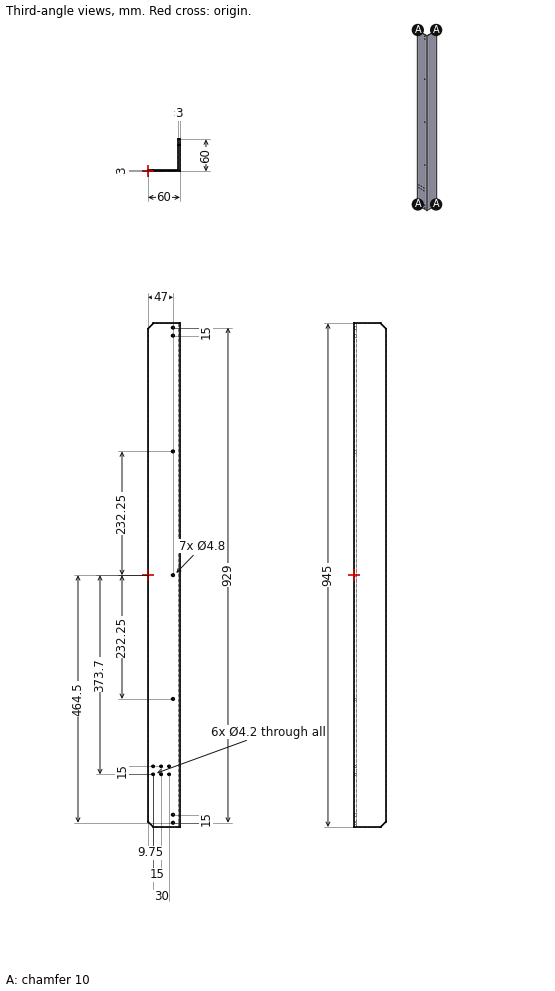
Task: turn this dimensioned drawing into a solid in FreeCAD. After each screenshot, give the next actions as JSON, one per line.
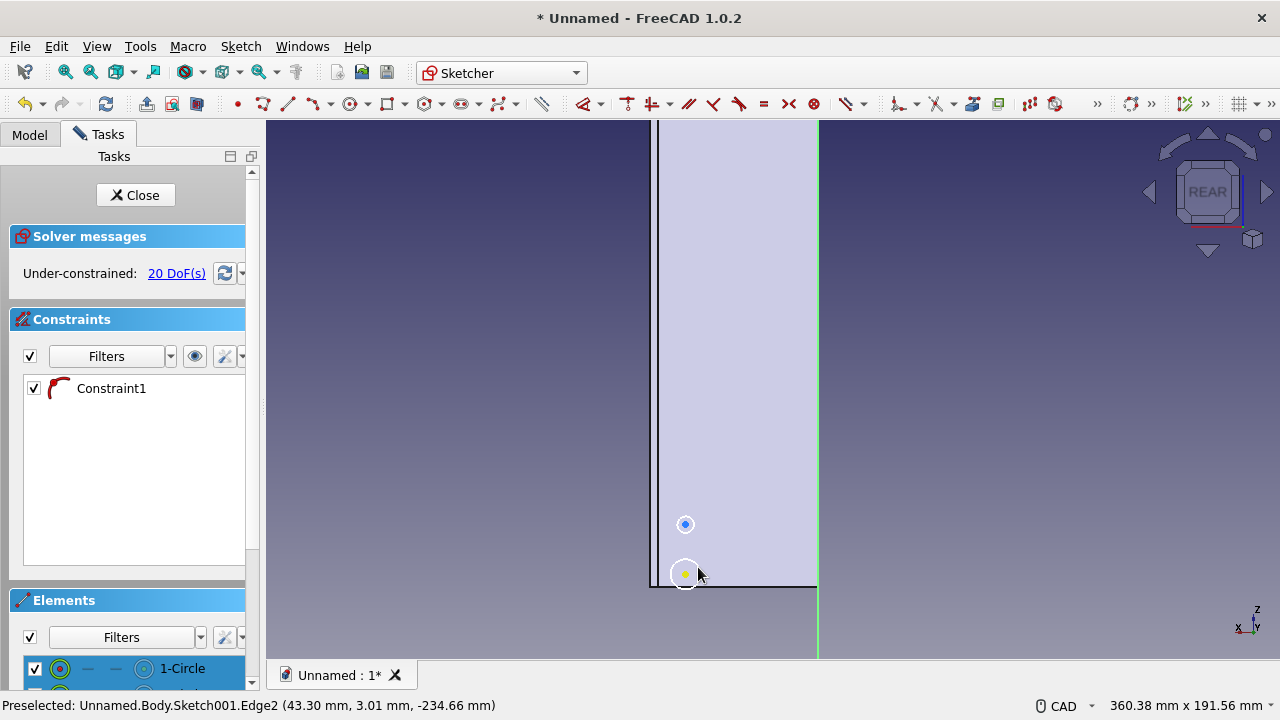
{"action": "left_click", "coordinate": [696, 564]}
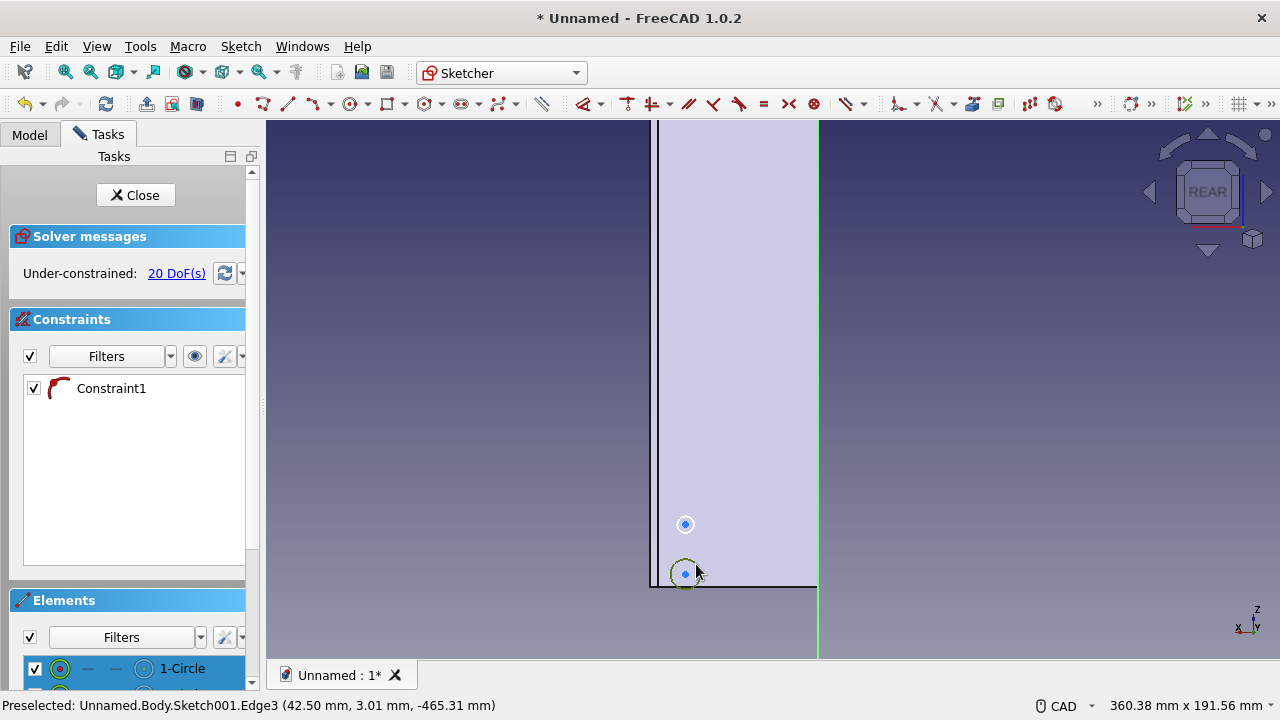
{"action": "scroll", "coordinate": [698, 567], "scroll_direction": "down", "scroll_amount": 10}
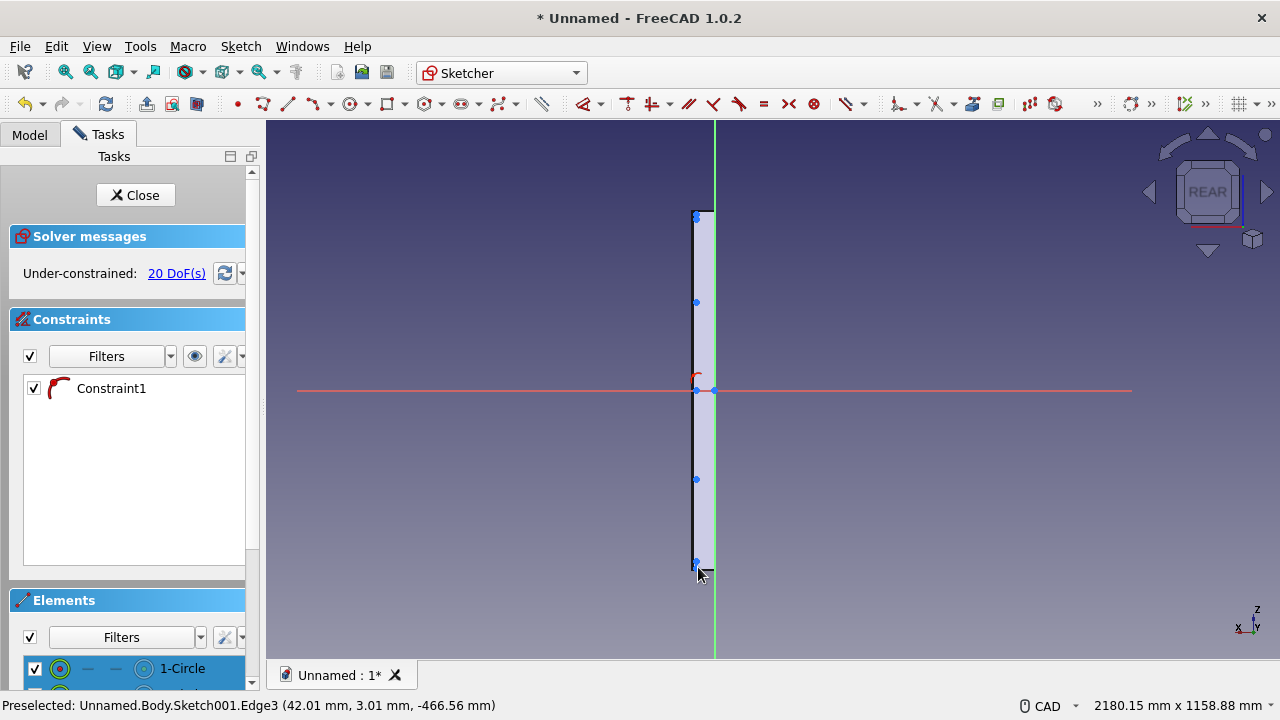
{"action": "scroll", "coordinate": [698, 213], "scroll_direction": "up", "scroll_amount": 11}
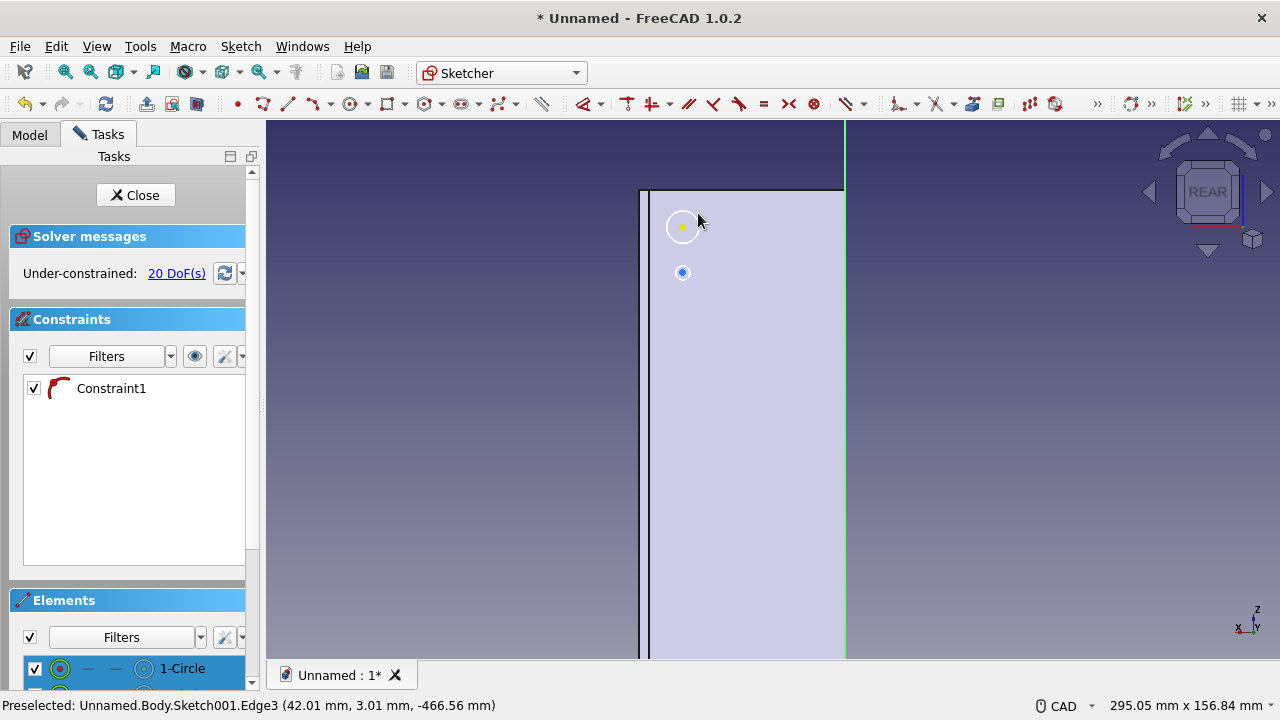
{"action": "left_click", "coordinate": [694, 216]}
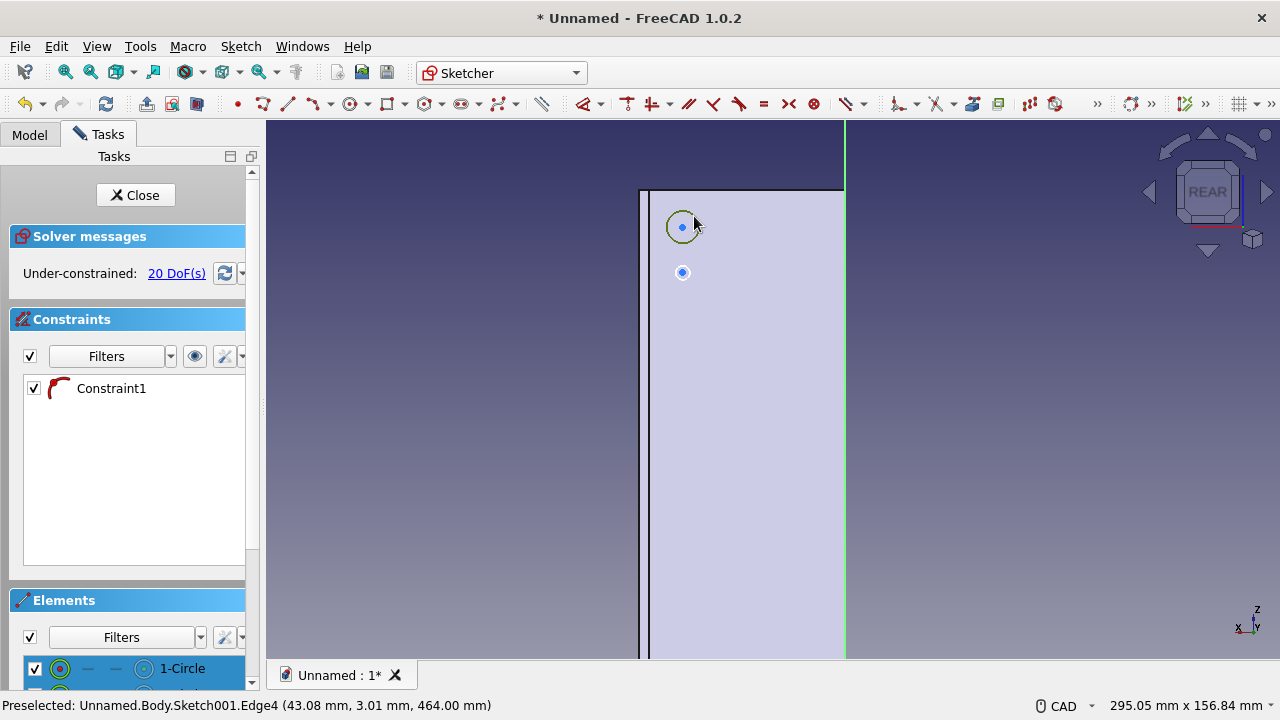
{"action": "scroll", "coordinate": [698, 212], "scroll_direction": "down", "scroll_amount": 11}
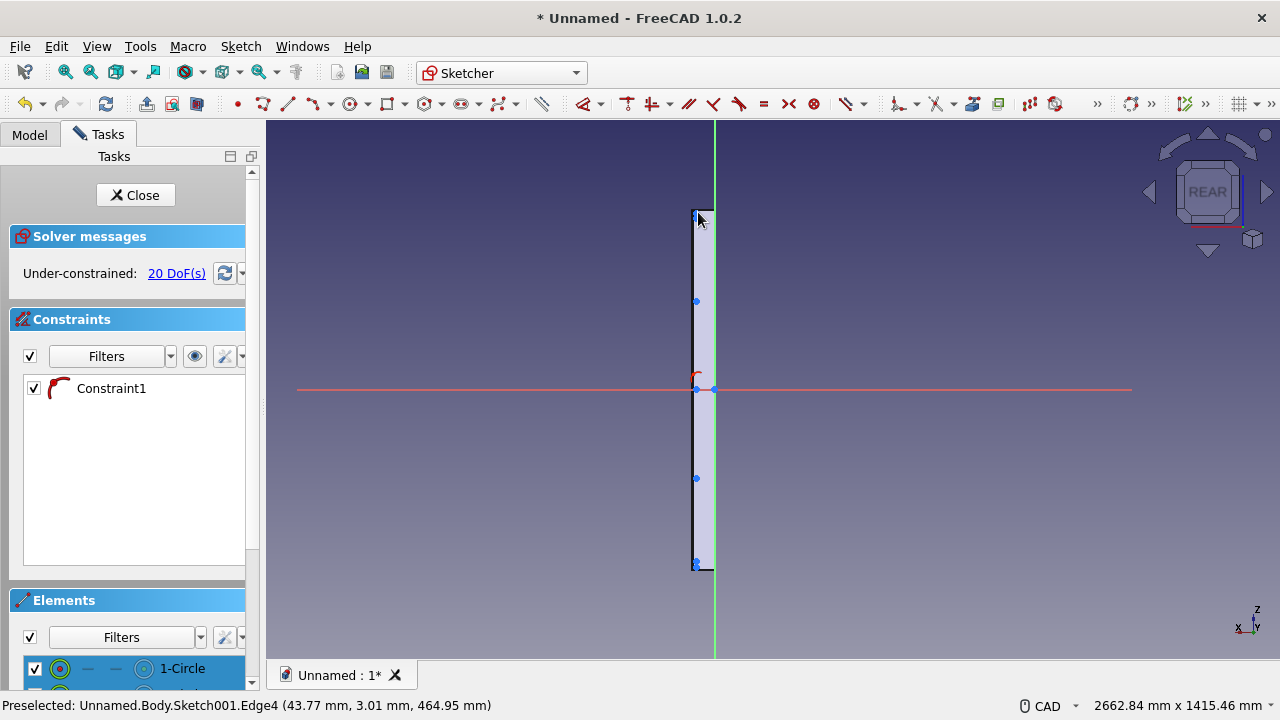
{"action": "scroll", "coordinate": [698, 301], "scroll_direction": "up", "scroll_amount": 12}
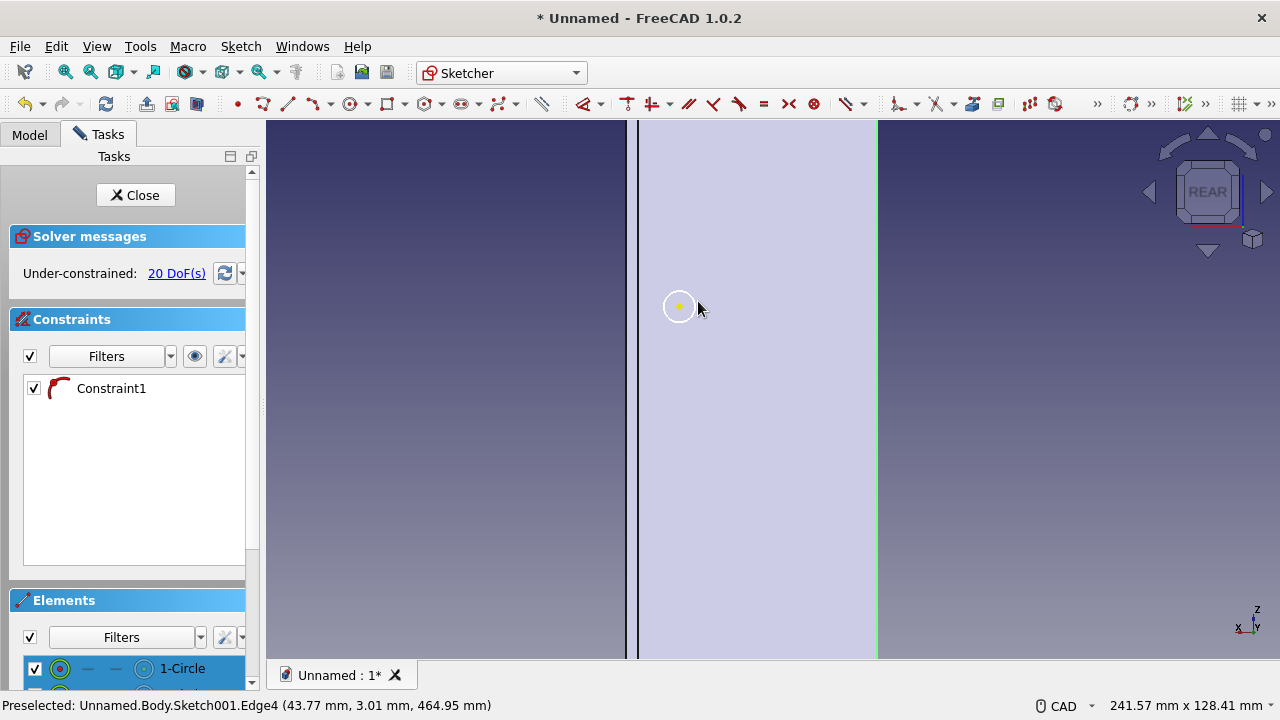
{"action": "left_click", "coordinate": [690, 296]}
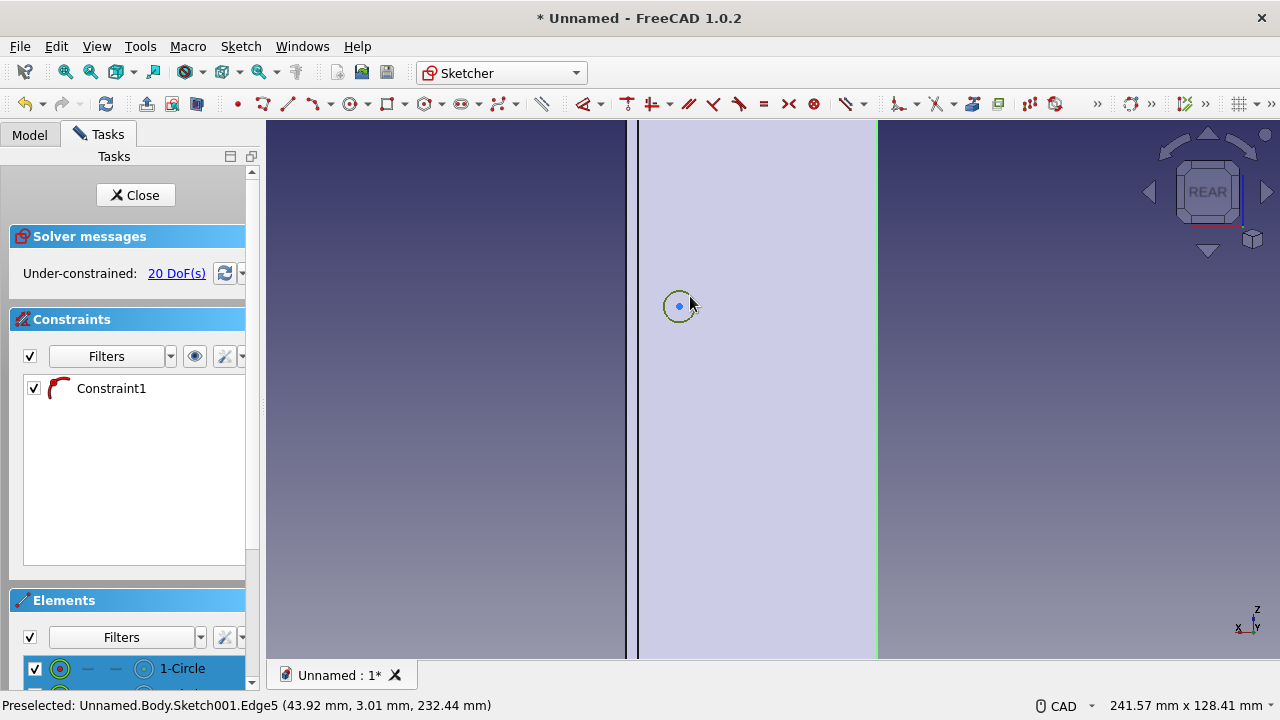
{"action": "scroll", "coordinate": [698, 301], "scroll_direction": "down", "scroll_amount": 12}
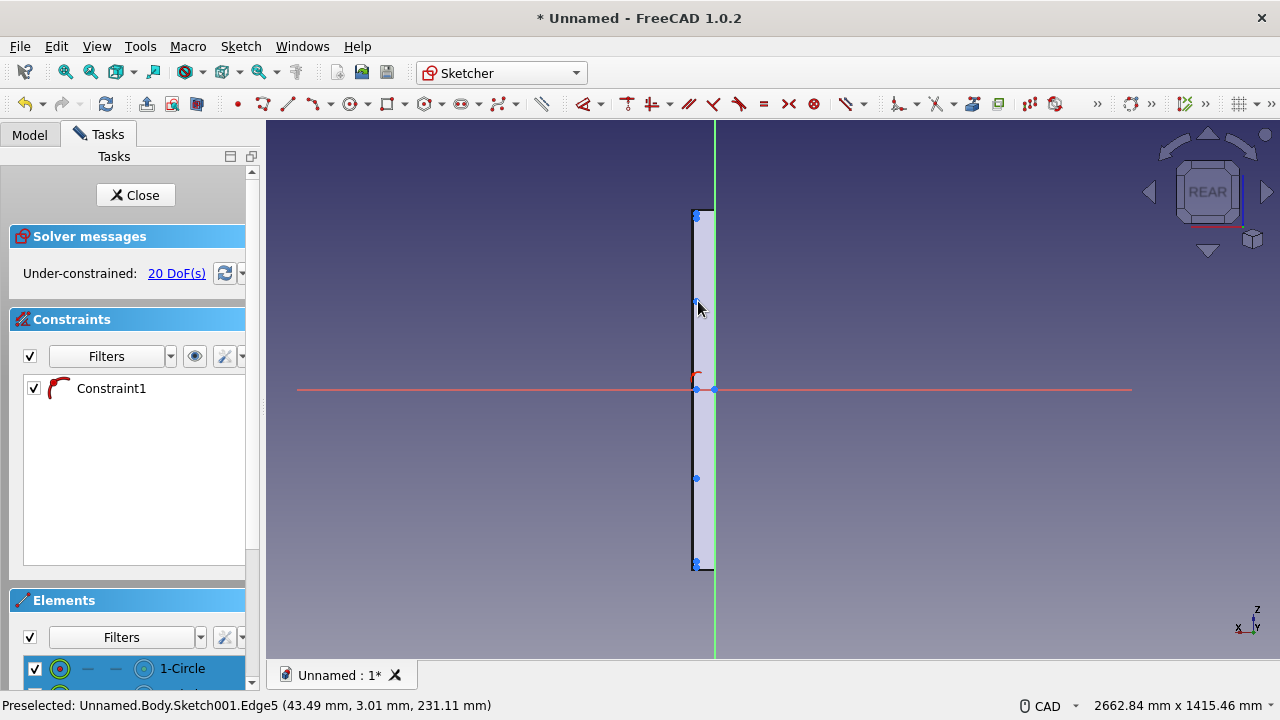
{"action": "scroll", "coordinate": [697, 560], "scroll_direction": "up", "scroll_amount": 13}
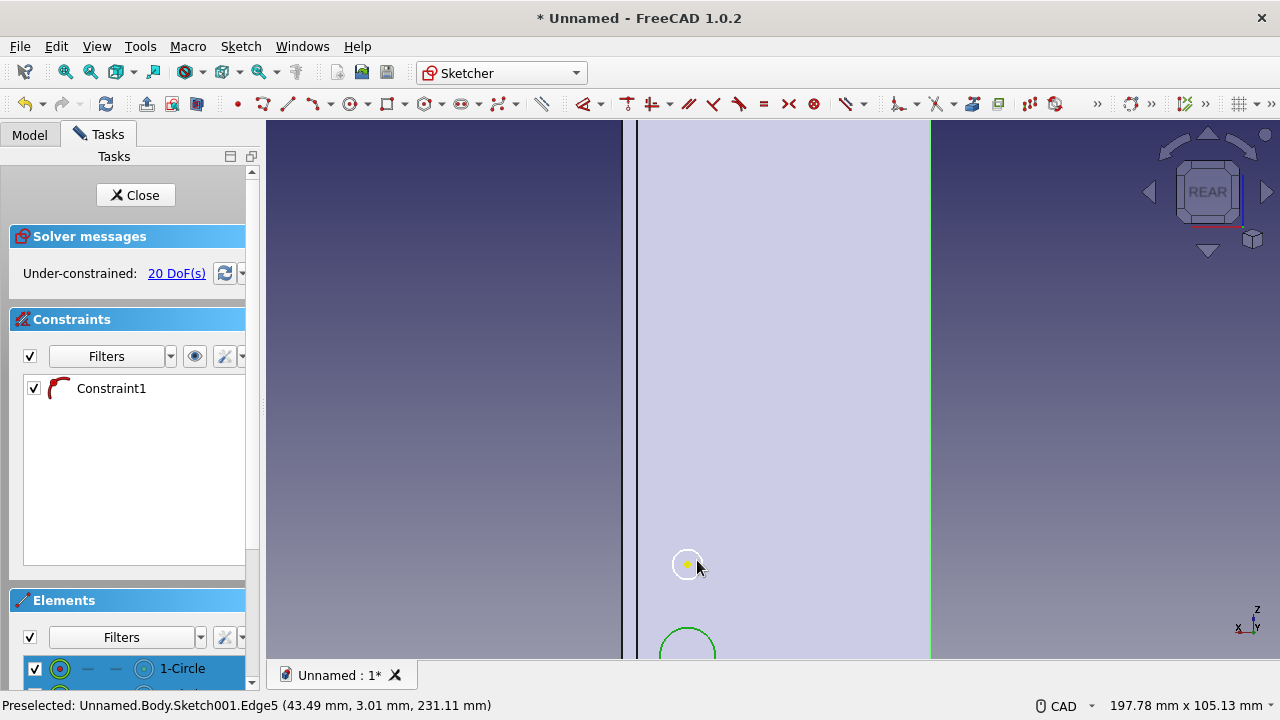
{"action": "left_click", "coordinate": [698, 554]}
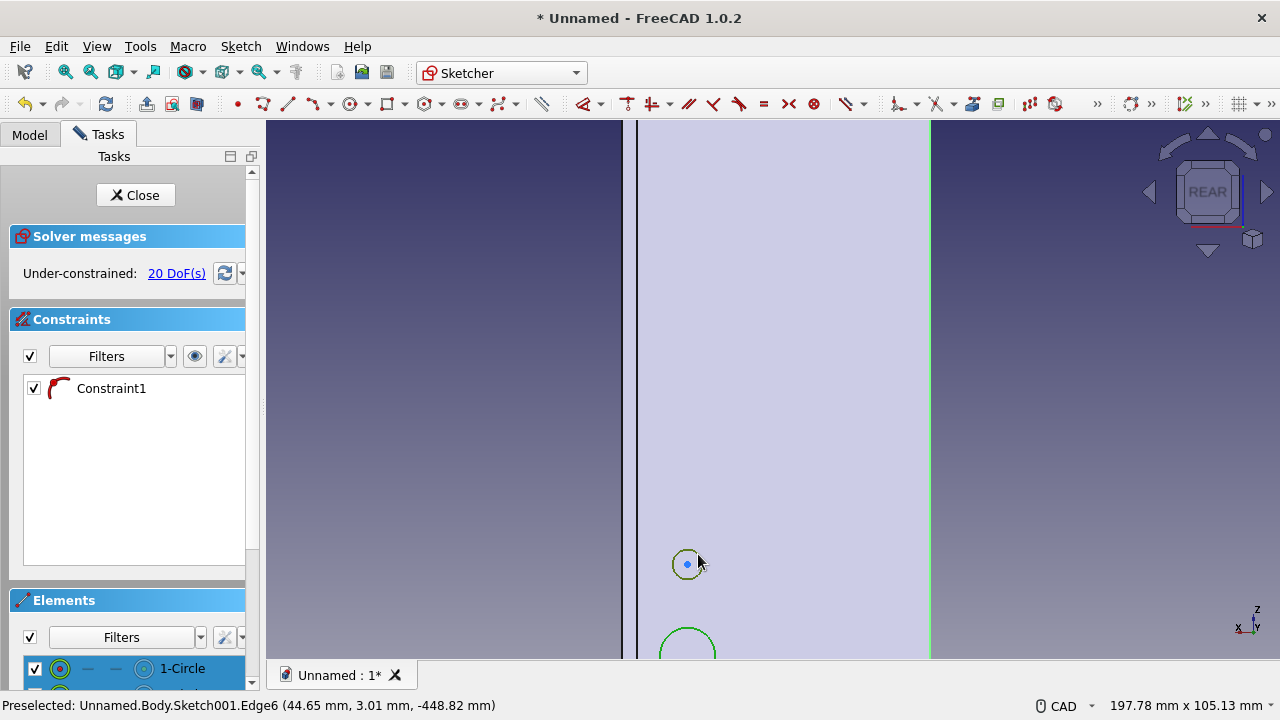
{"action": "scroll", "coordinate": [697, 561], "scroll_direction": "down", "scroll_amount": 13}